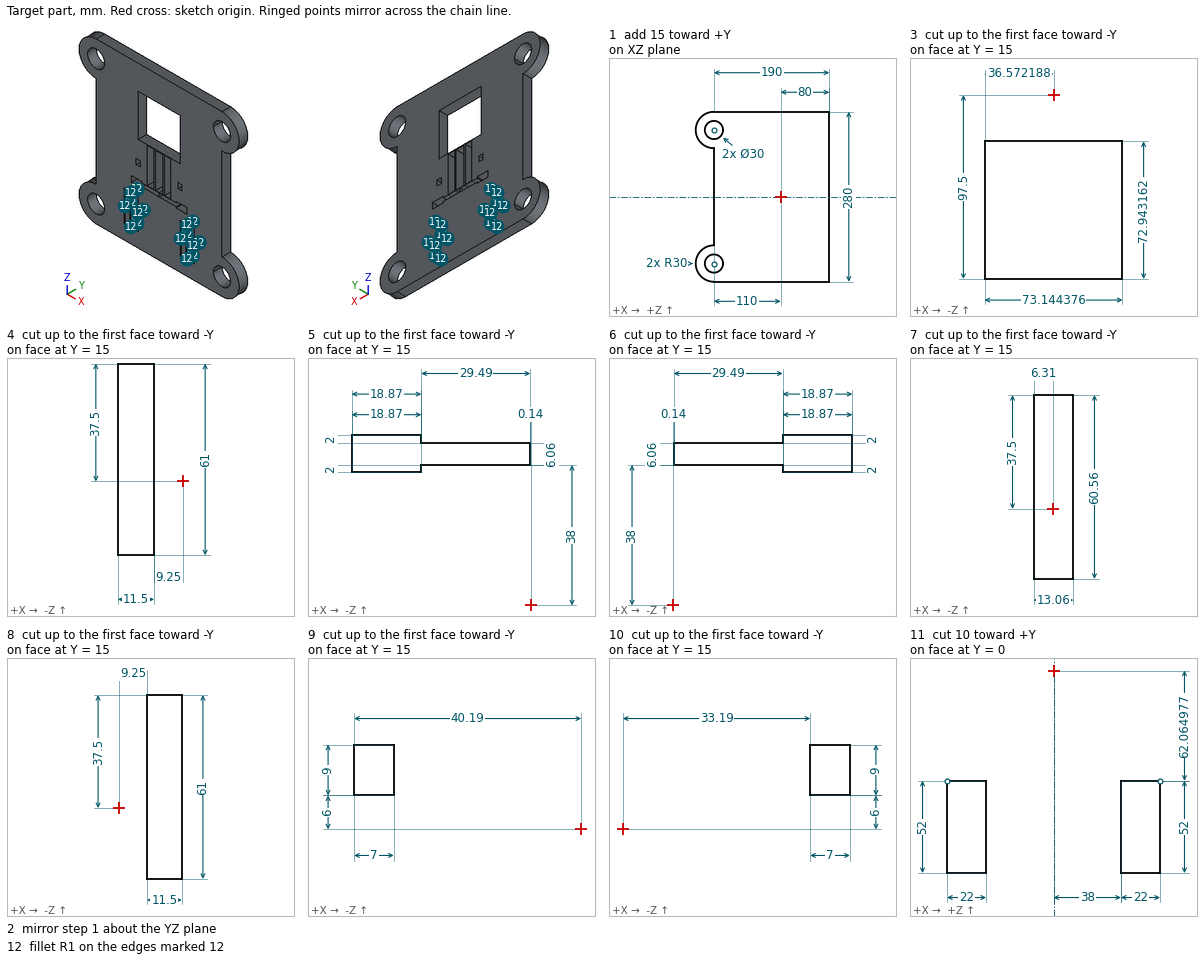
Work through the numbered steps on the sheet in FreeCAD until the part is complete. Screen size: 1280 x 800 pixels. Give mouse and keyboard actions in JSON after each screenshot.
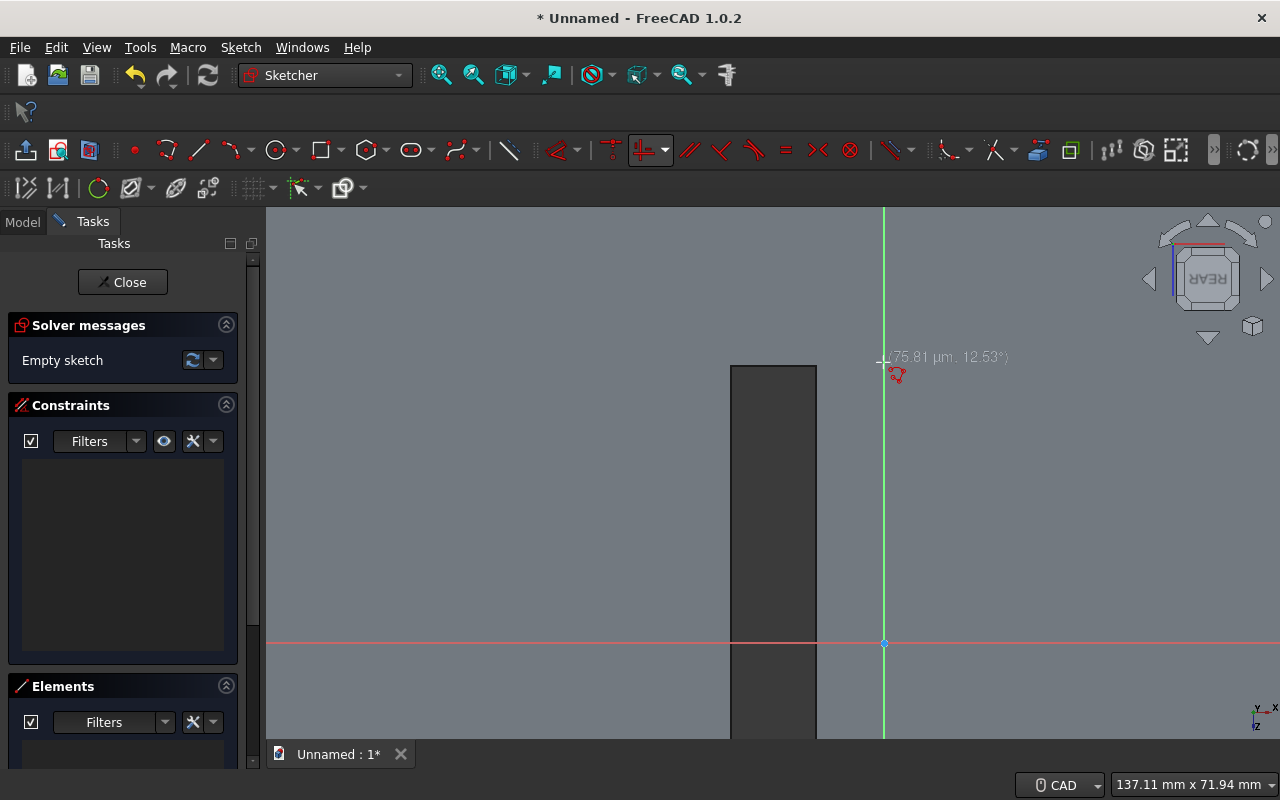
{"action": "scroll", "coordinate": [883, 317], "scroll_direction": "up", "scroll_amount": 14}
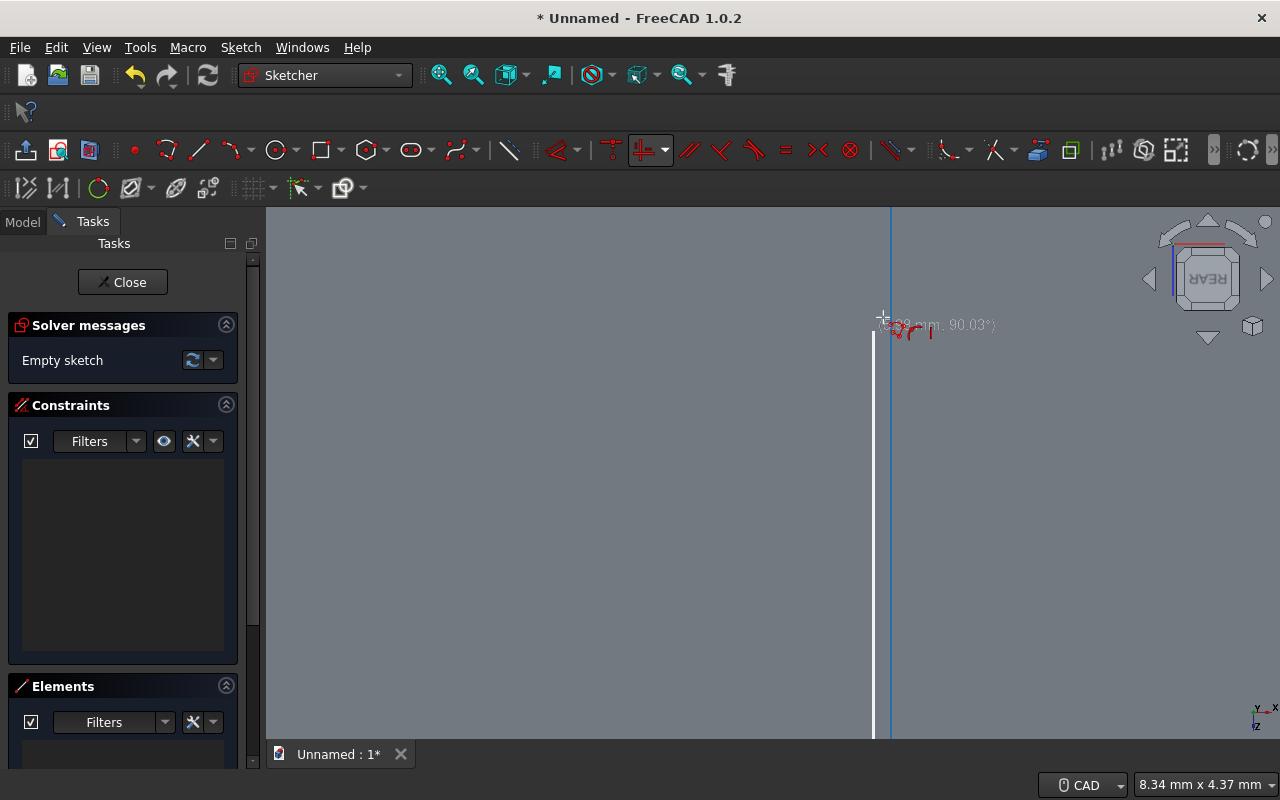
{"action": "left_click", "coordinate": [874, 320]}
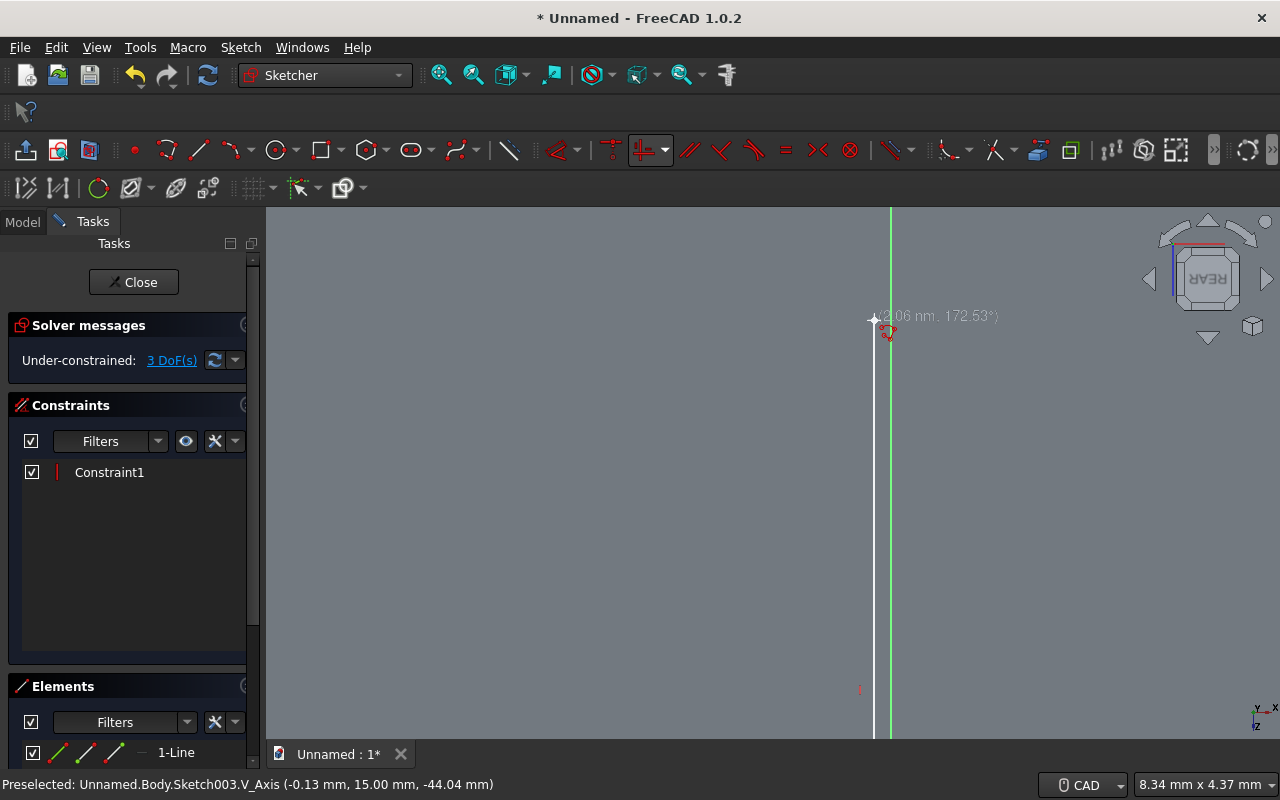
{"action": "scroll", "coordinate": [883, 317], "scroll_direction": "down", "scroll_amount": 14}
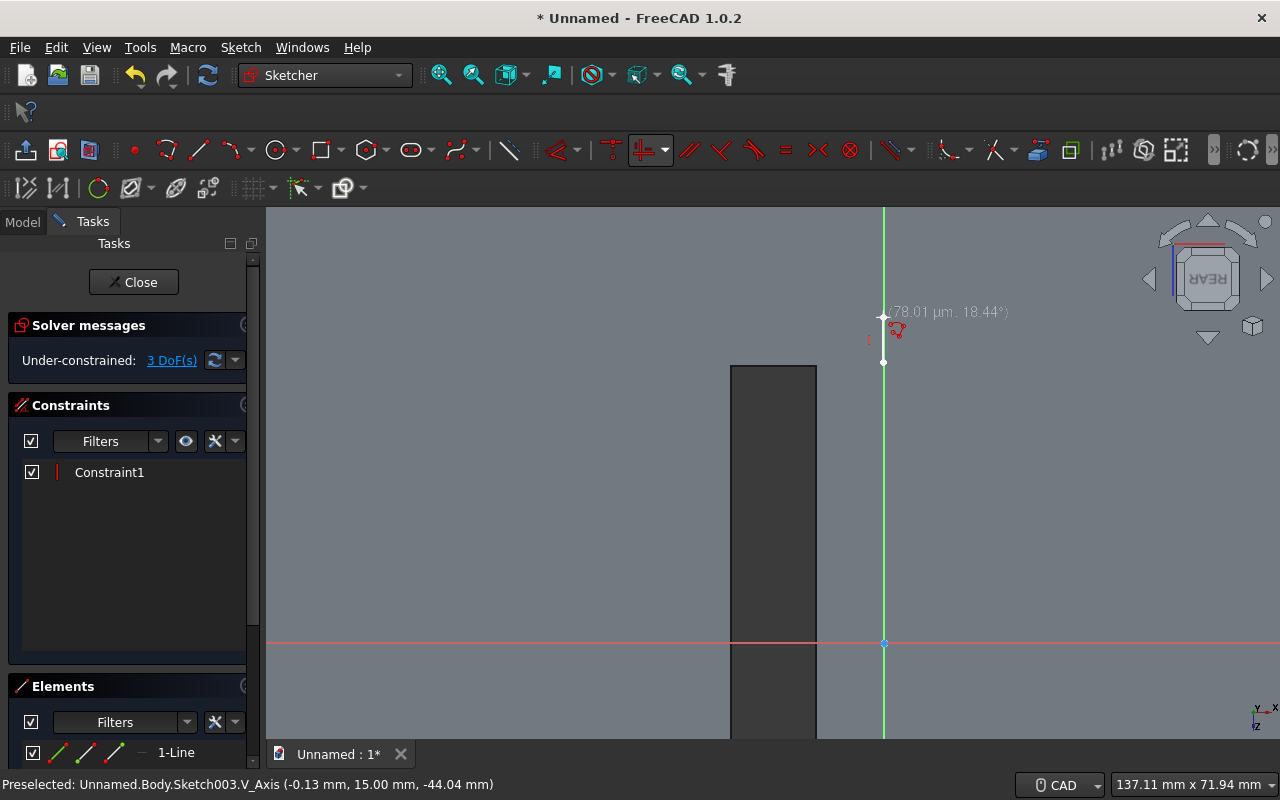
{"action": "left_click", "coordinate": [665, 317]}
{"action": "left_click", "coordinate": [665, 303]}
{"action": "left_click", "coordinate": [525, 303]}
{"action": "left_click", "coordinate": [525, 377]}
{"action": "left_click", "coordinate": [665, 377]}
{"action": "left_click", "coordinate": [665, 362]}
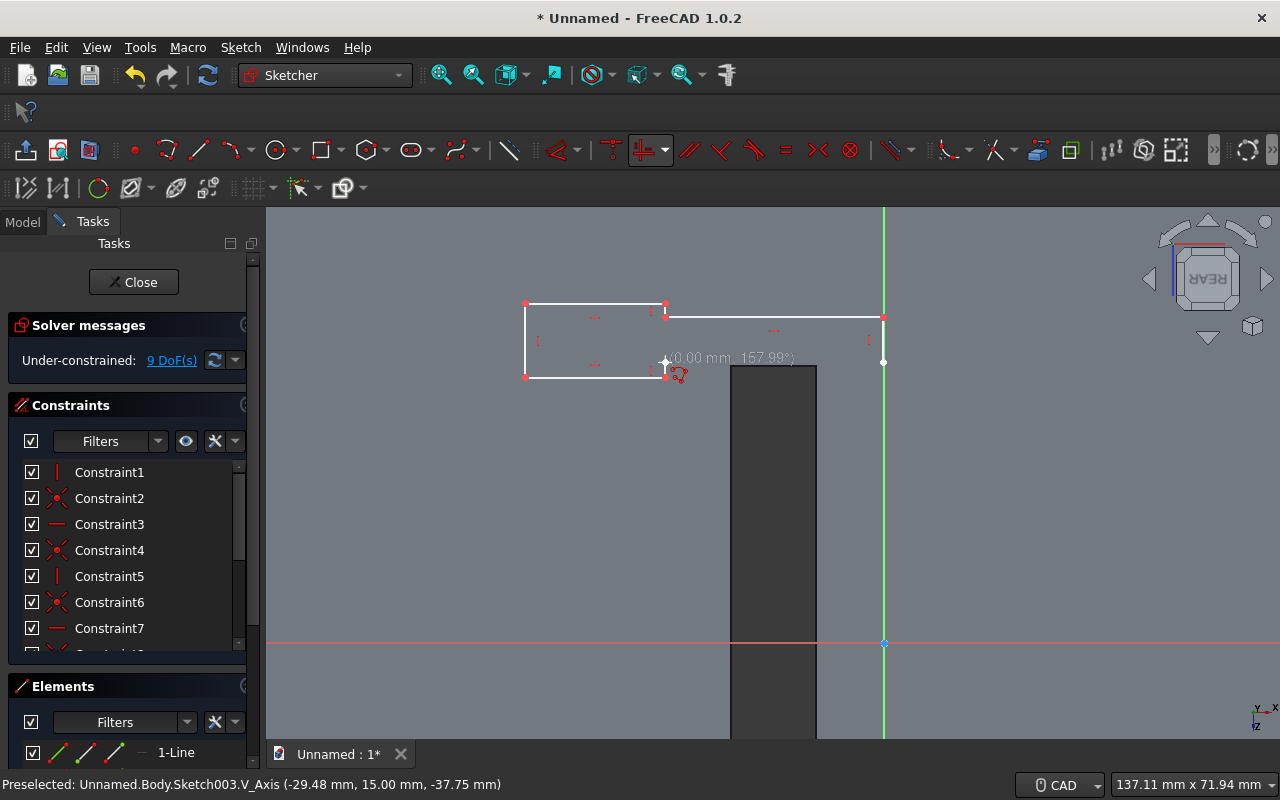
{"action": "scroll", "coordinate": [883, 362], "scroll_direction": "up", "scroll_amount": 14}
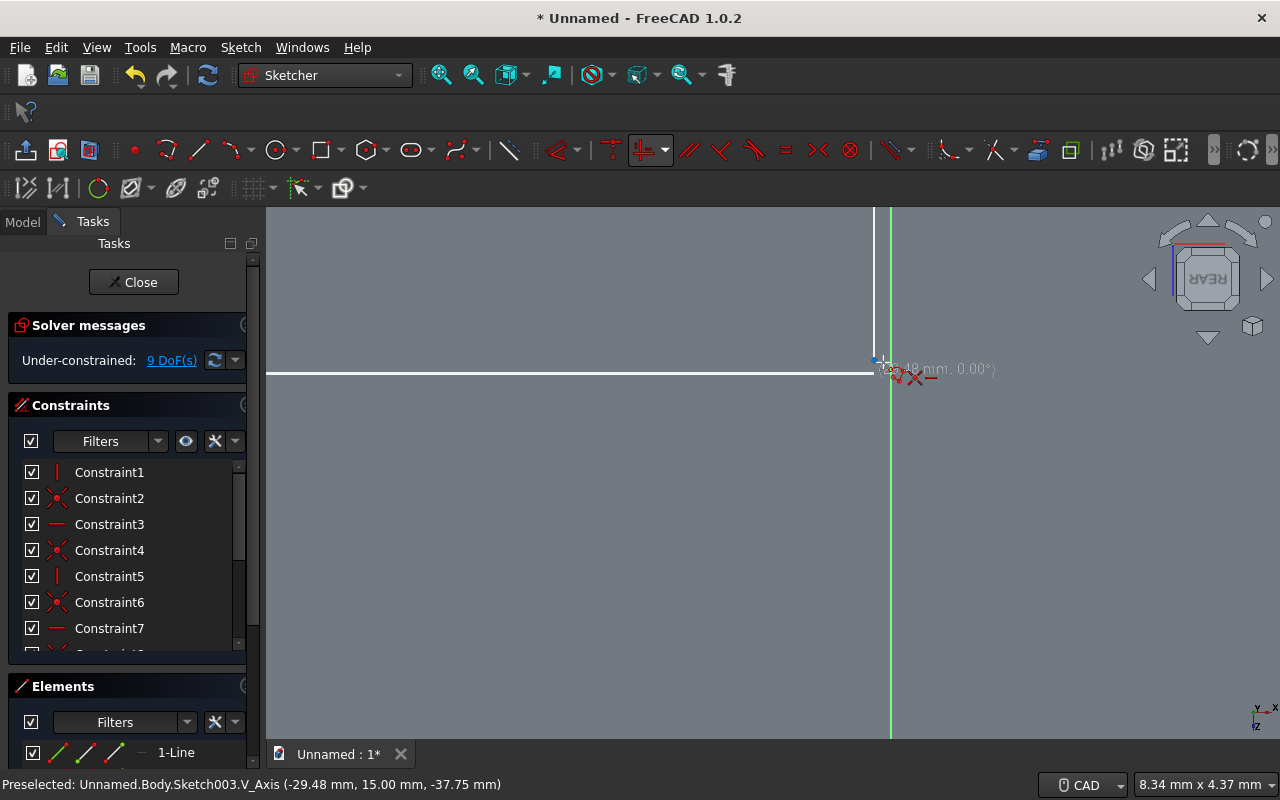
{"action": "left_click", "coordinate": [874, 361]}
{"action": "key", "text": "Escape"}
{"action": "key", "text": "Escape"}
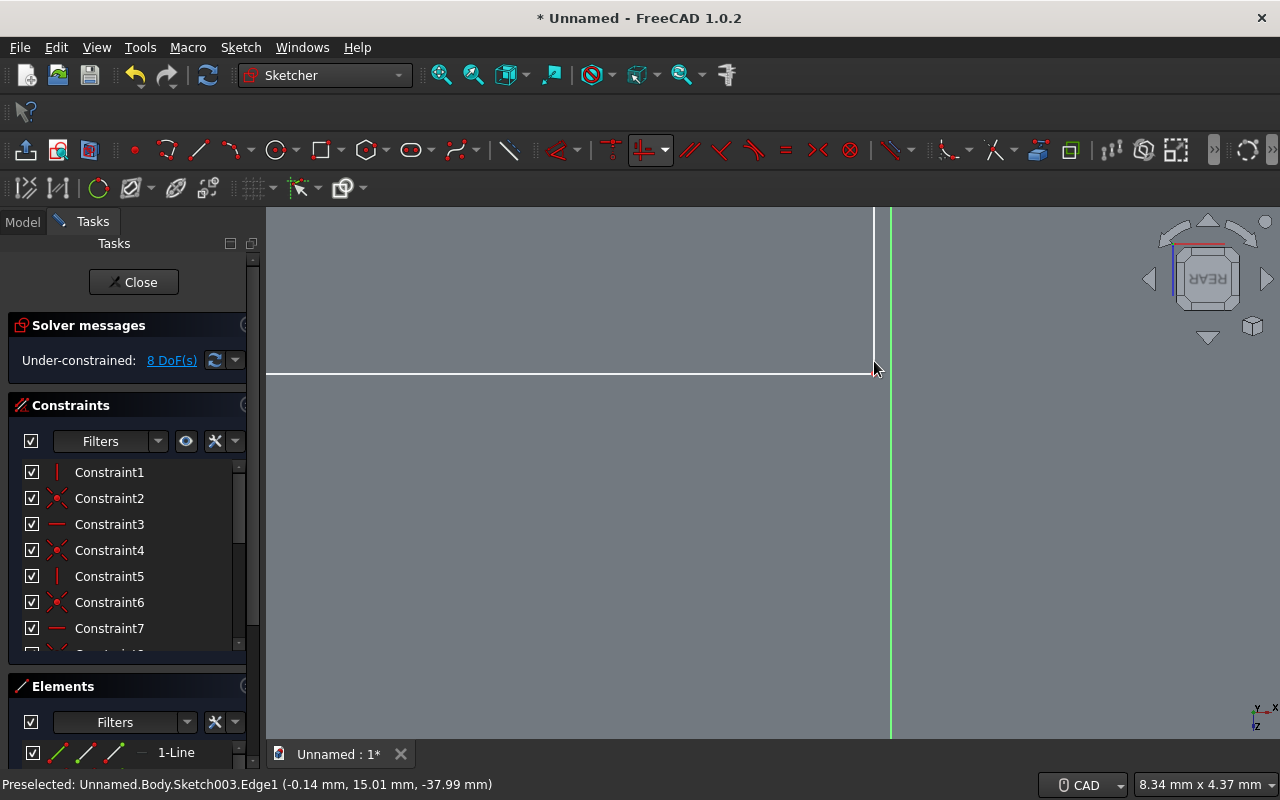
{"action": "key", "text": "d"}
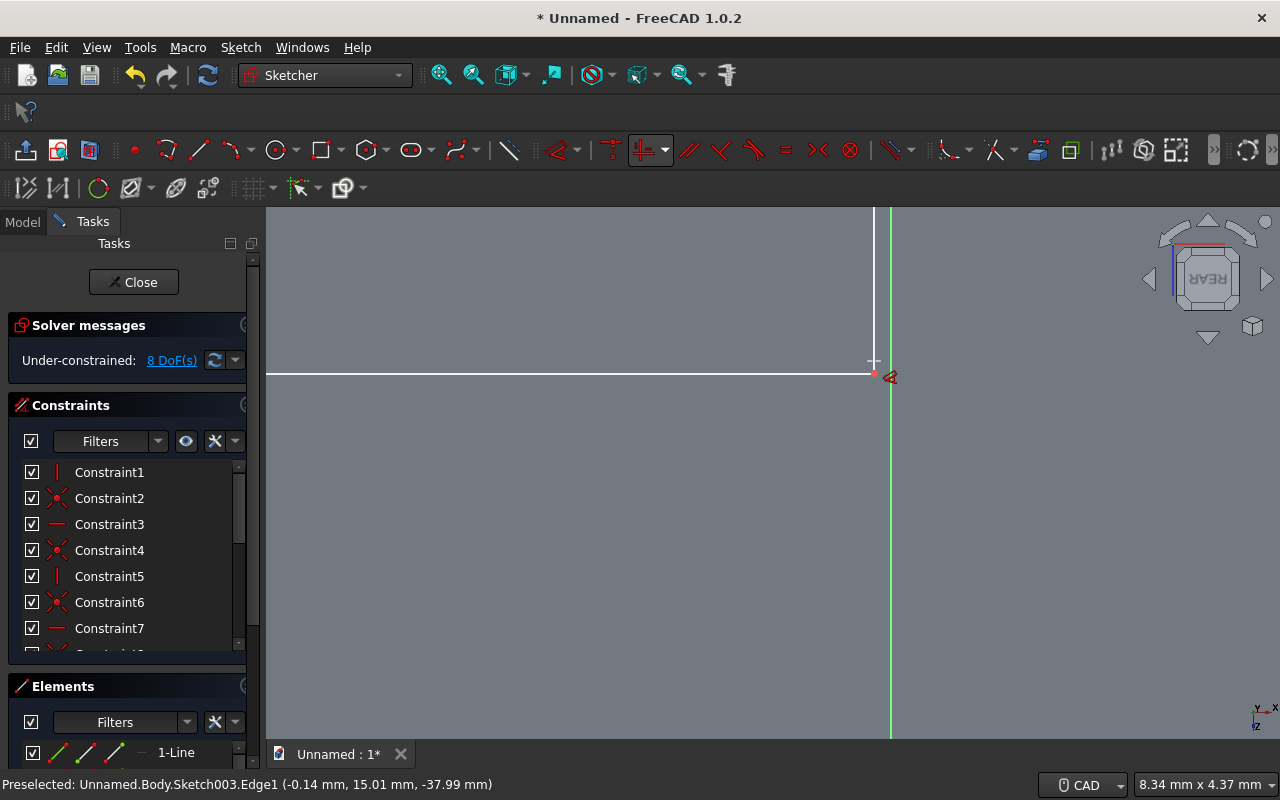
{"action": "scroll", "coordinate": [883, 362], "scroll_direction": "down", "scroll_amount": 14}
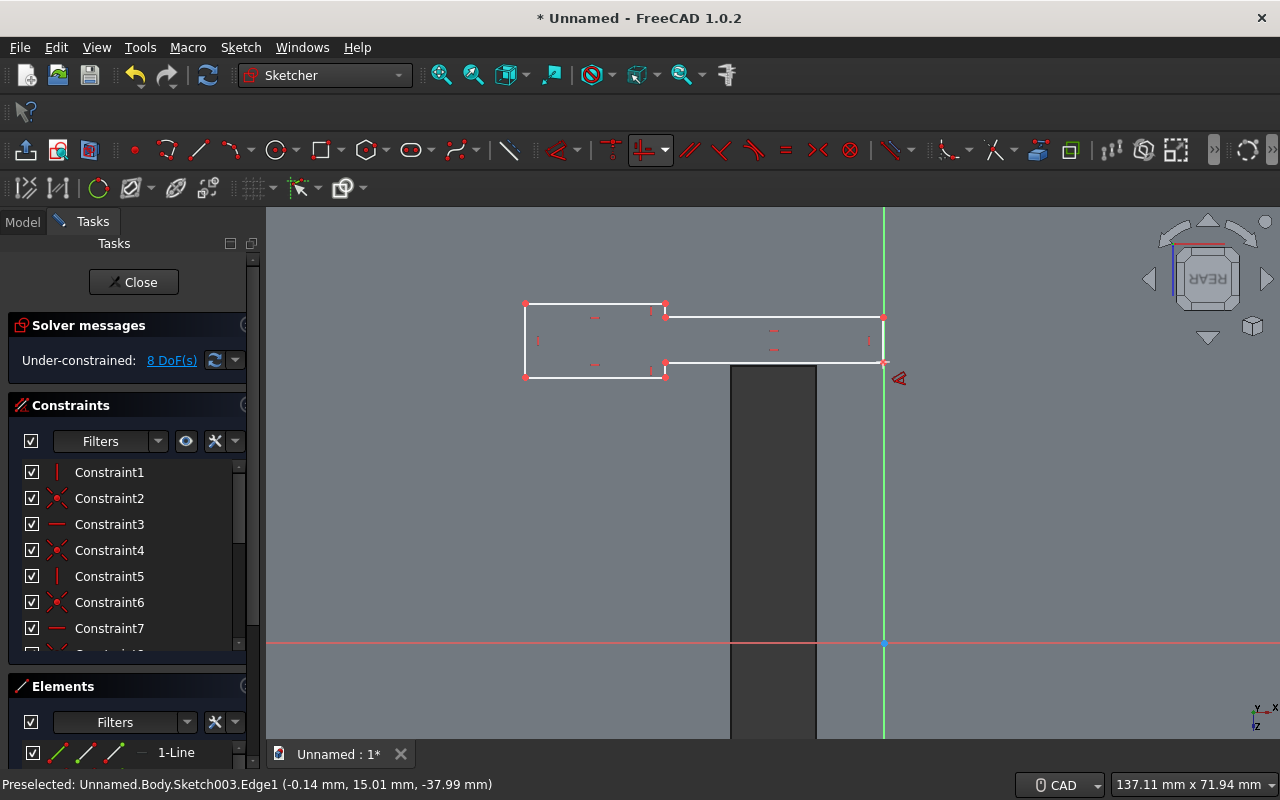
{"action": "scroll", "coordinate": [665, 313], "scroll_direction": "up", "scroll_amount": 7}